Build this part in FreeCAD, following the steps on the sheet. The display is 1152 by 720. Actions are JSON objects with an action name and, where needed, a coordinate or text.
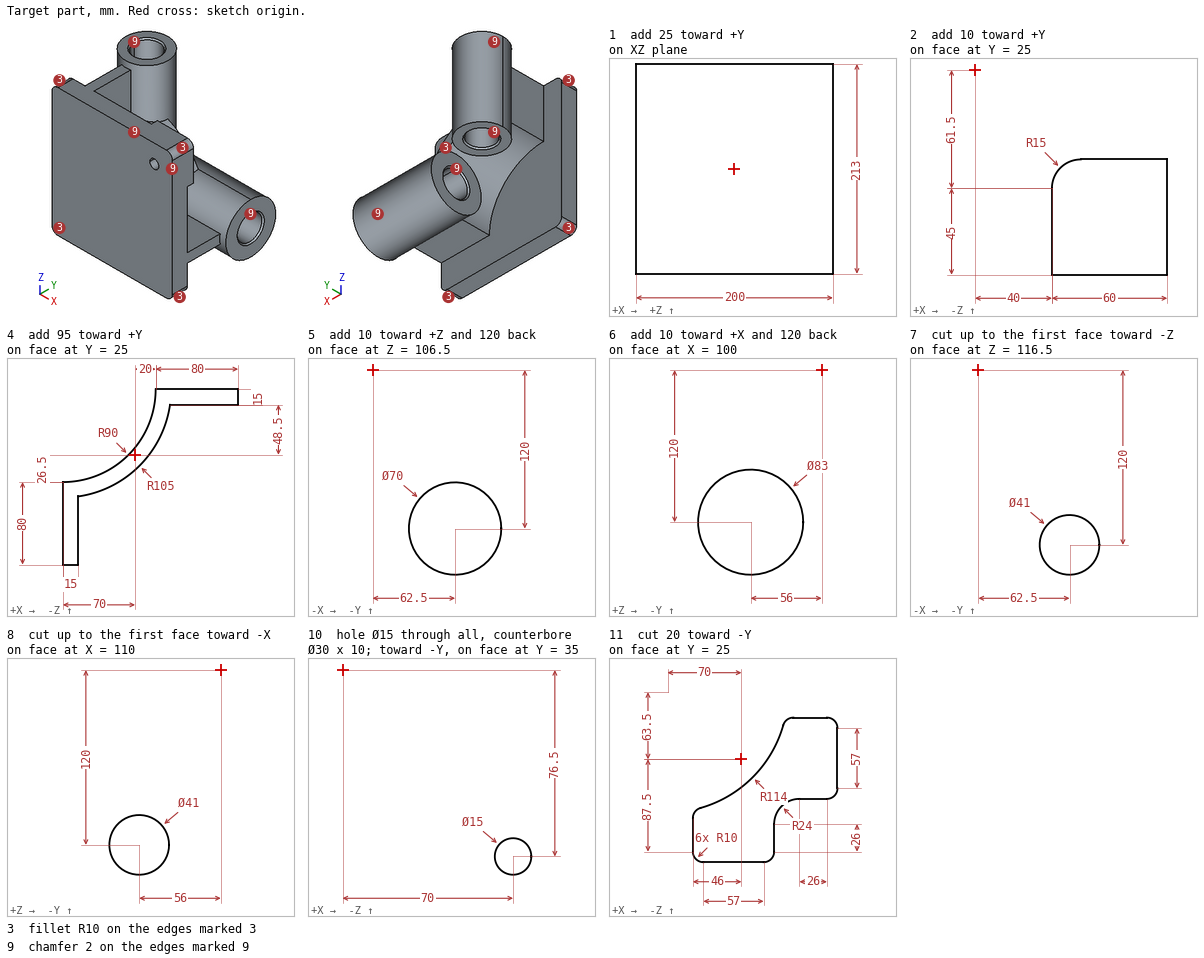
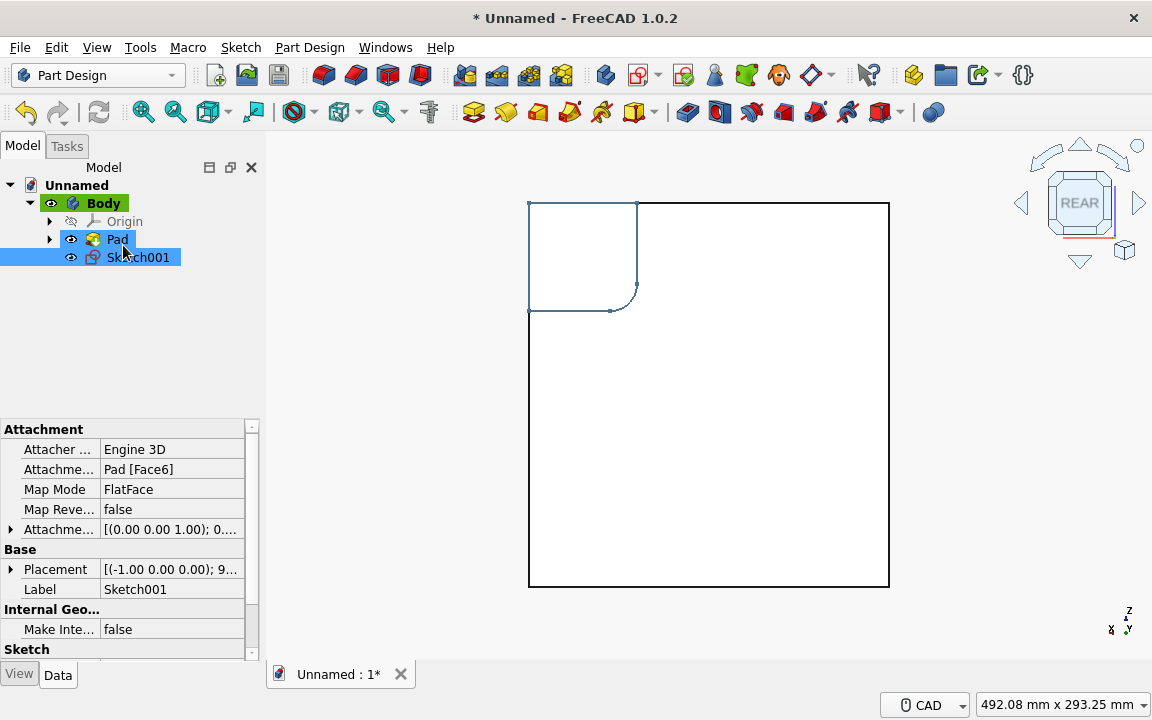
{"action": "left_click", "coordinate": [474, 112]}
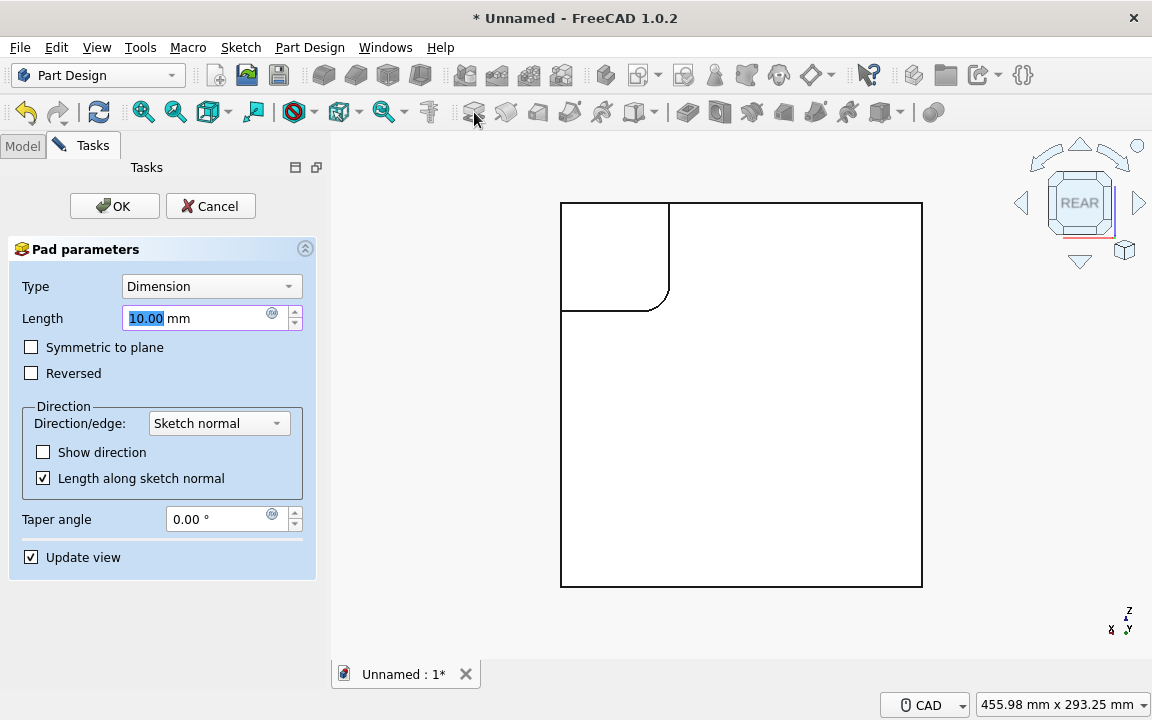
{"action": "type", "text": "10"}
{"action": "key", "text": "Tab"}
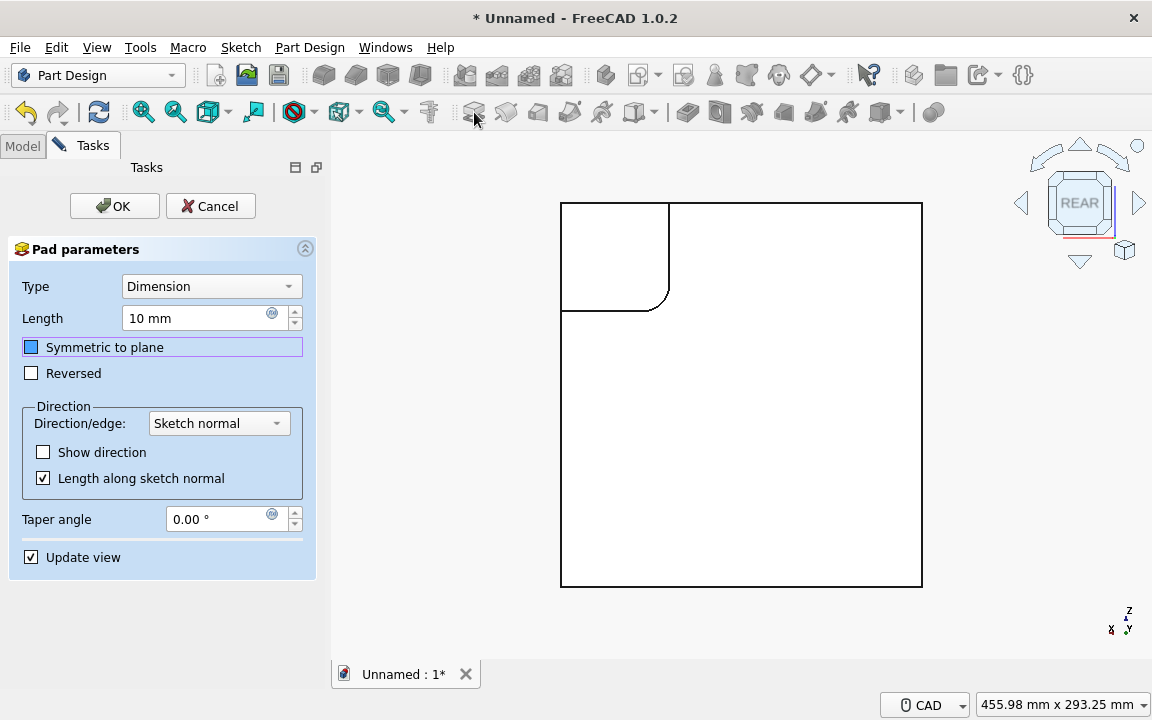
{"action": "left_click", "coordinate": [115, 206]}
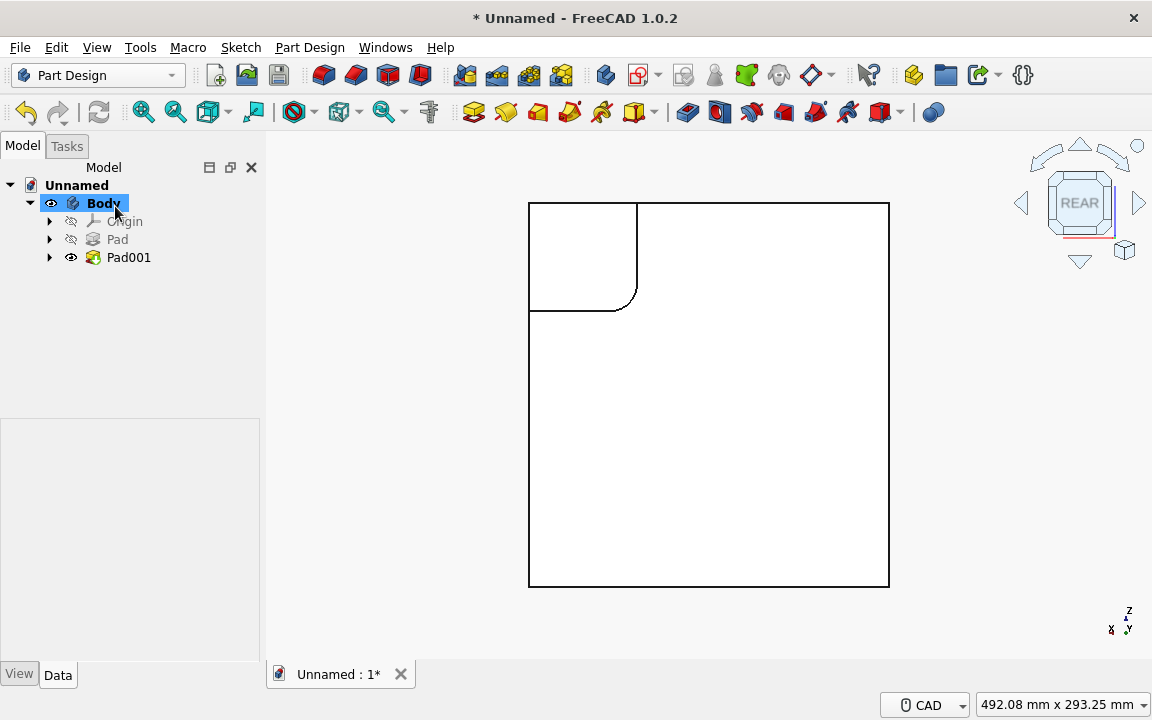
{"action": "key", "text": "0"}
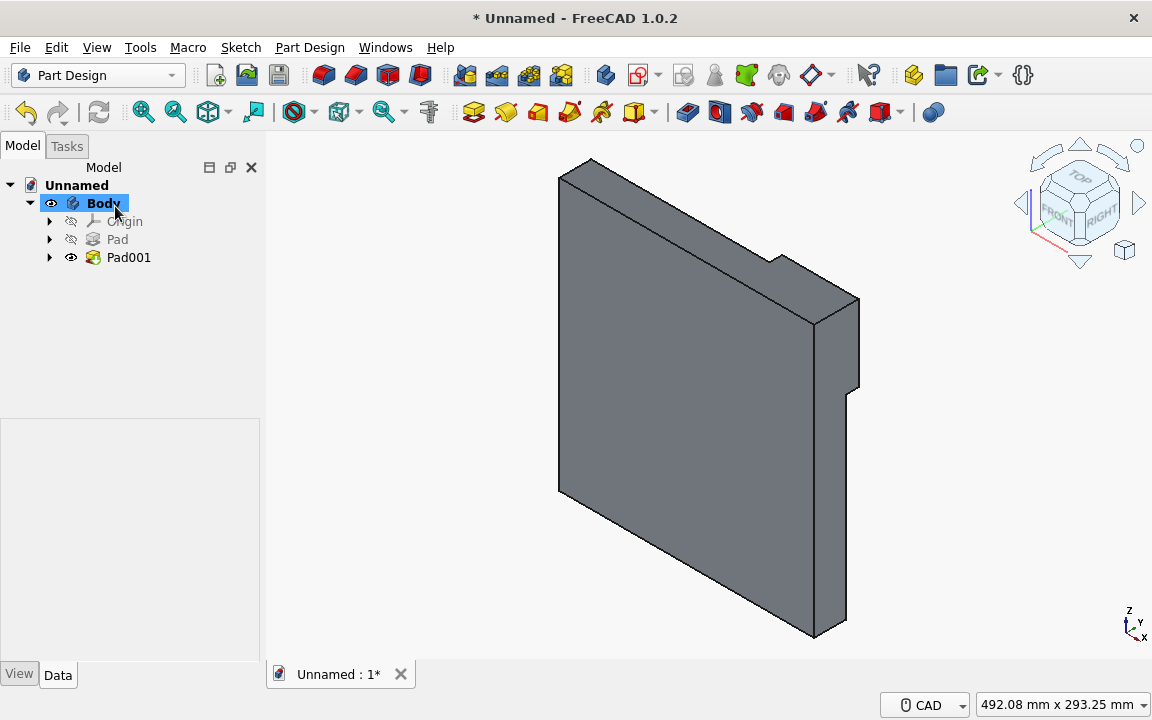
{"action": "left_click", "coordinate": [836, 311]}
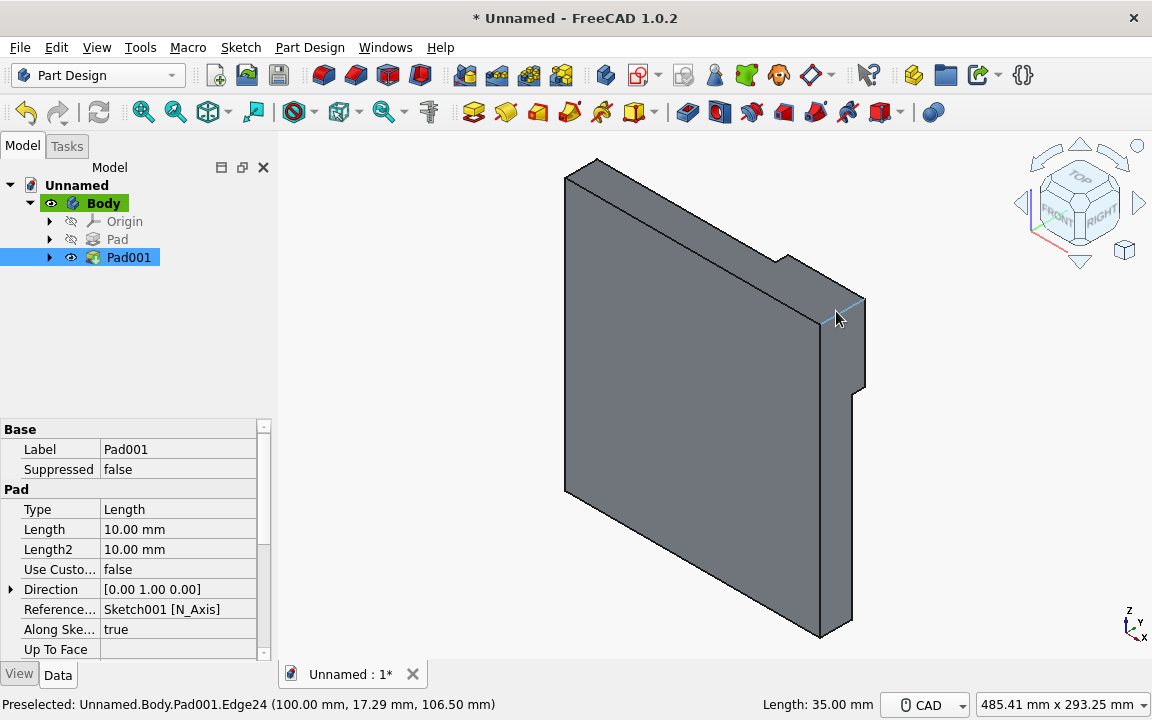
{"action": "key", "text": "2"}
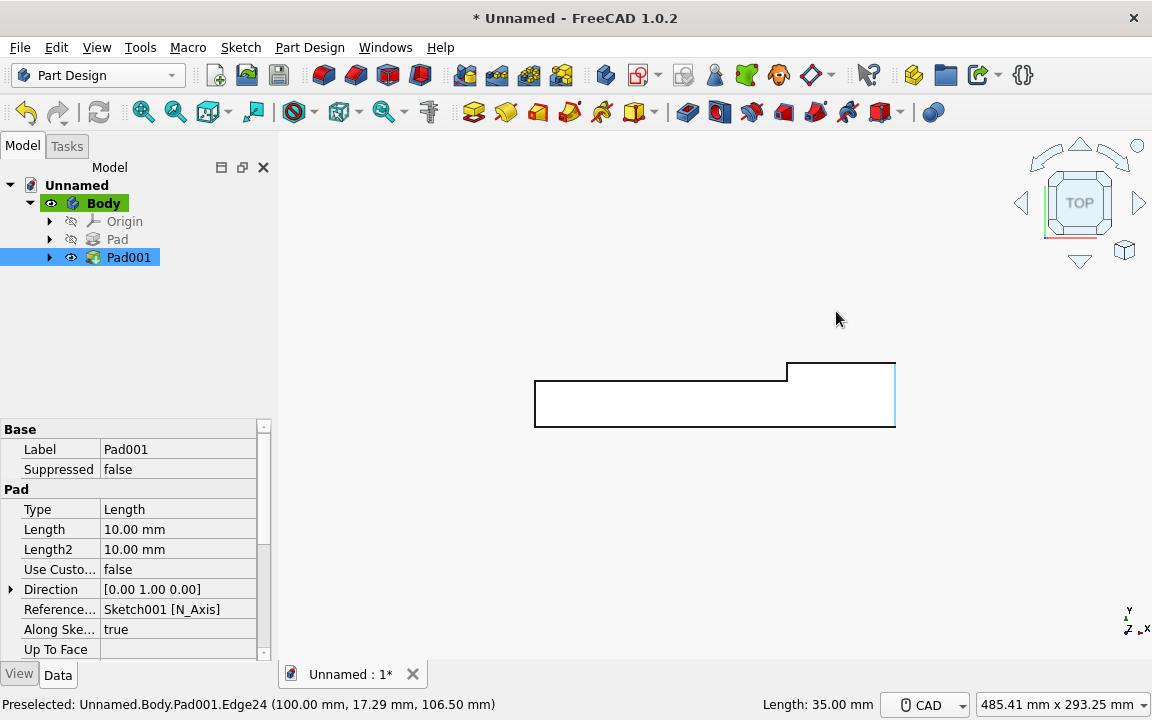
{"action": "left_click", "coordinate": [144, 112]}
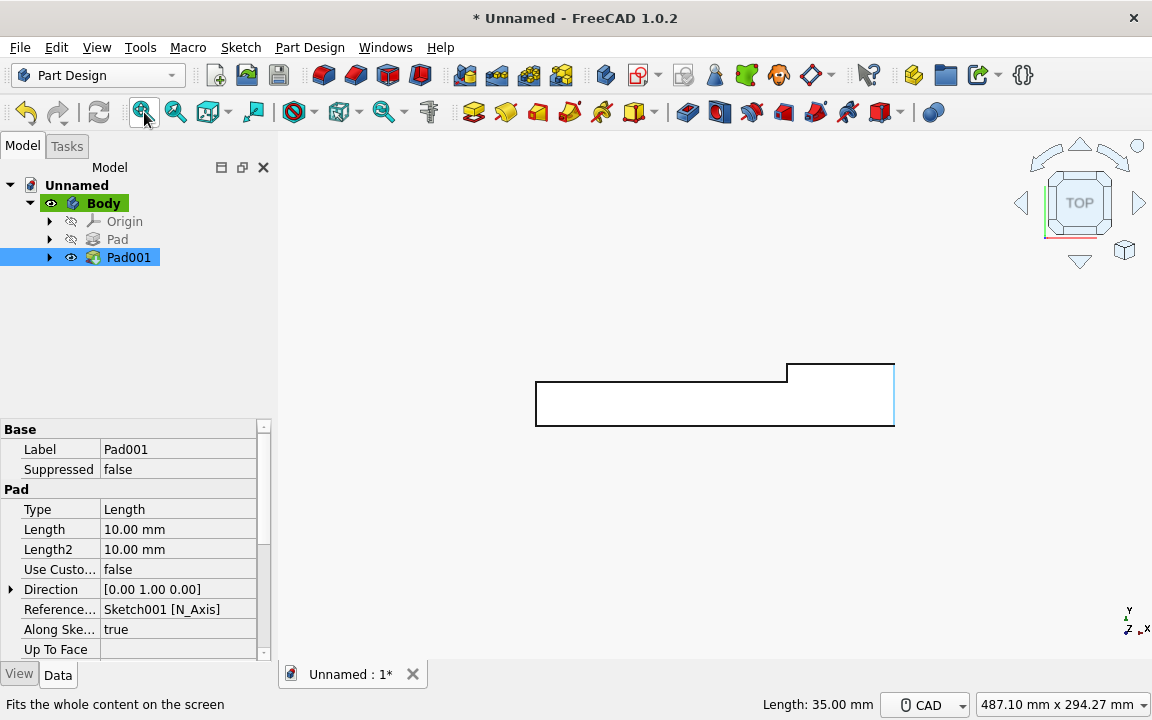
{"action": "left_click", "coordinate": [536, 403], "text": "ctrl"}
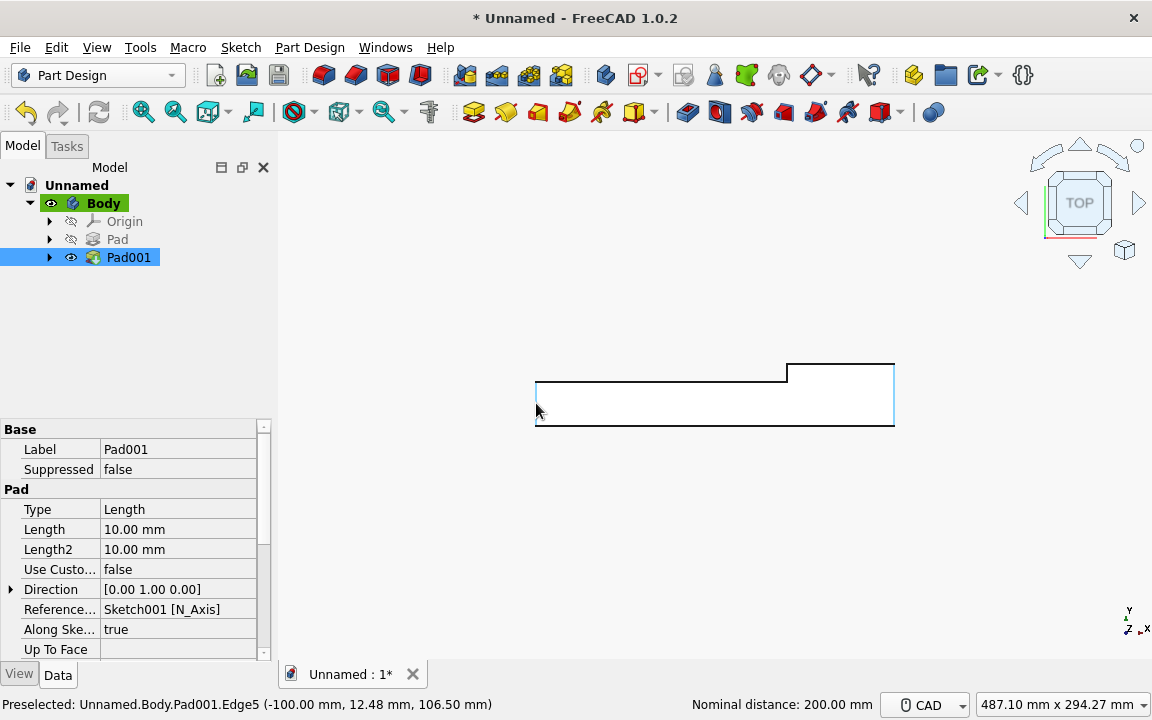
{"action": "key", "text": "1"}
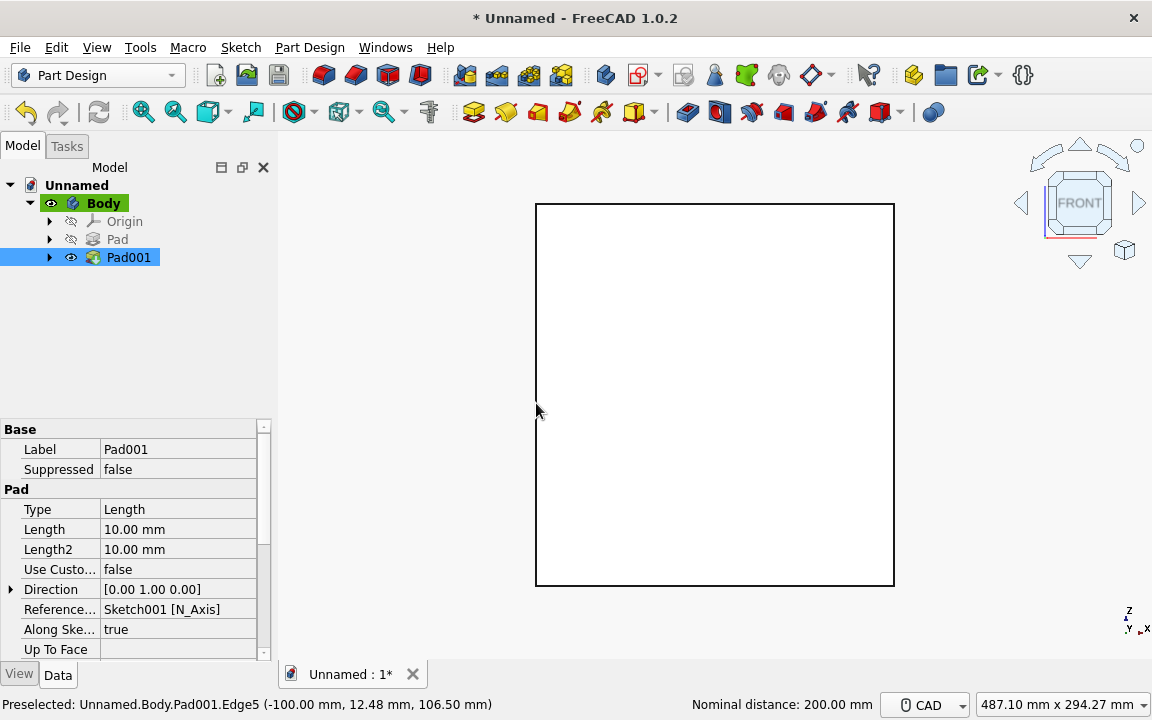
{"action": "key", "text": "3"}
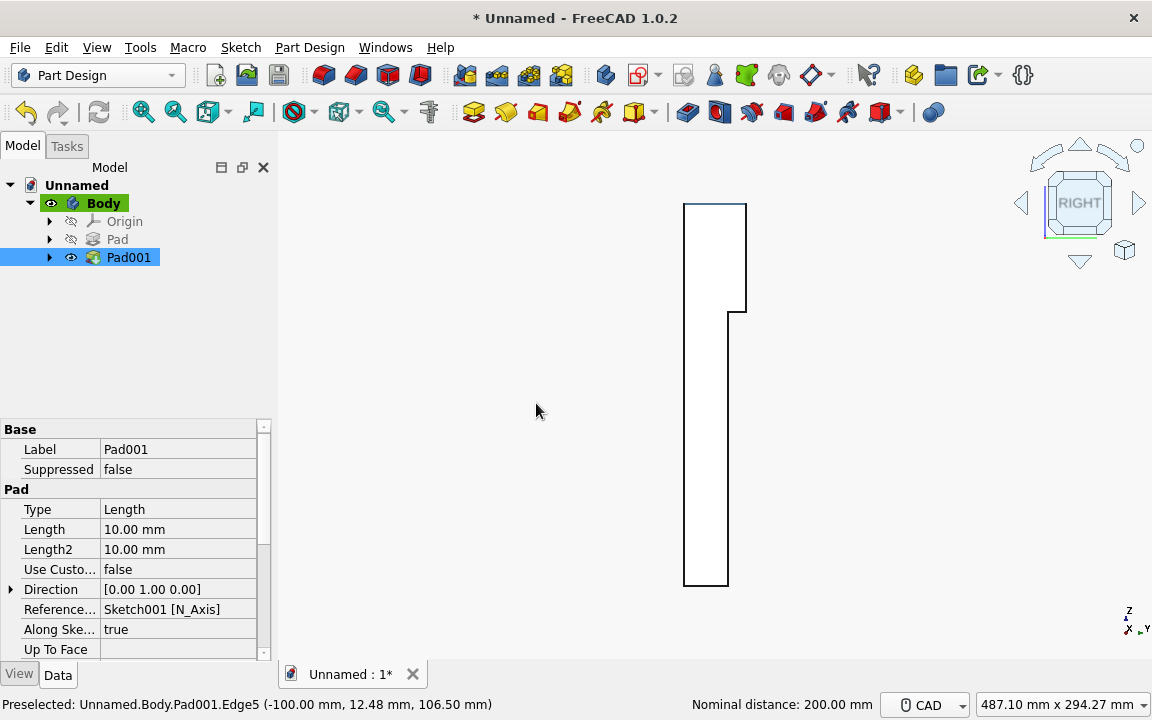
{"action": "left_click", "coordinate": [706, 585], "text": "ctrl"}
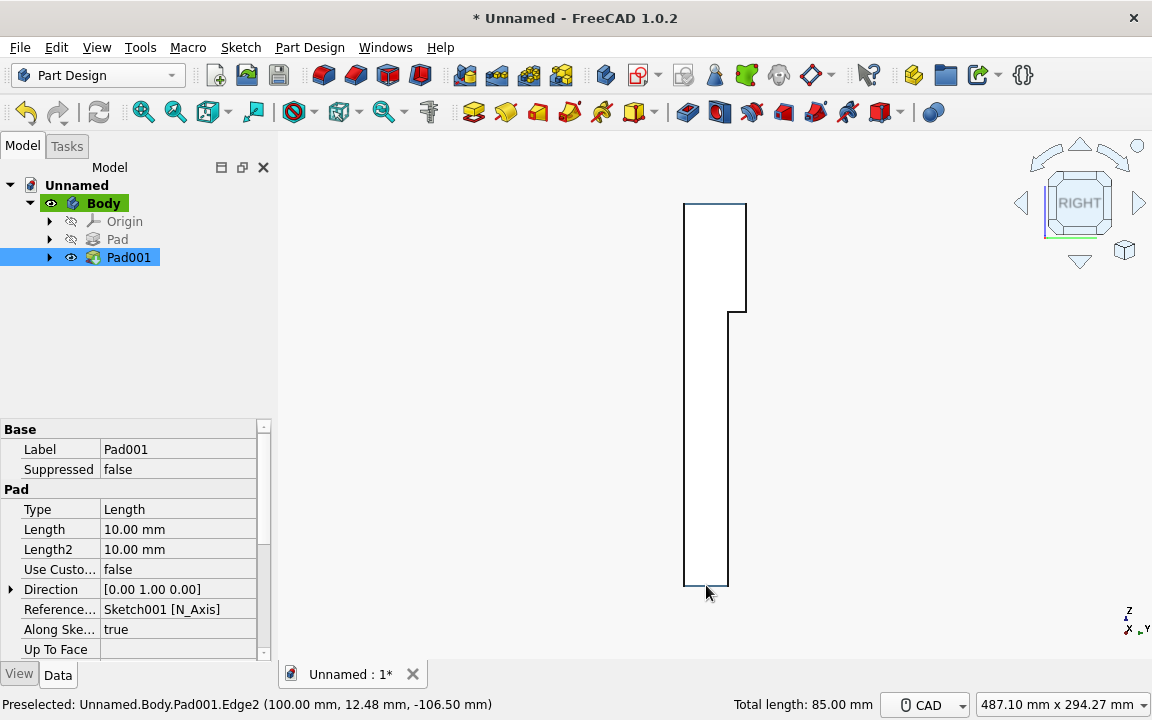
{"action": "key", "text": "5"}